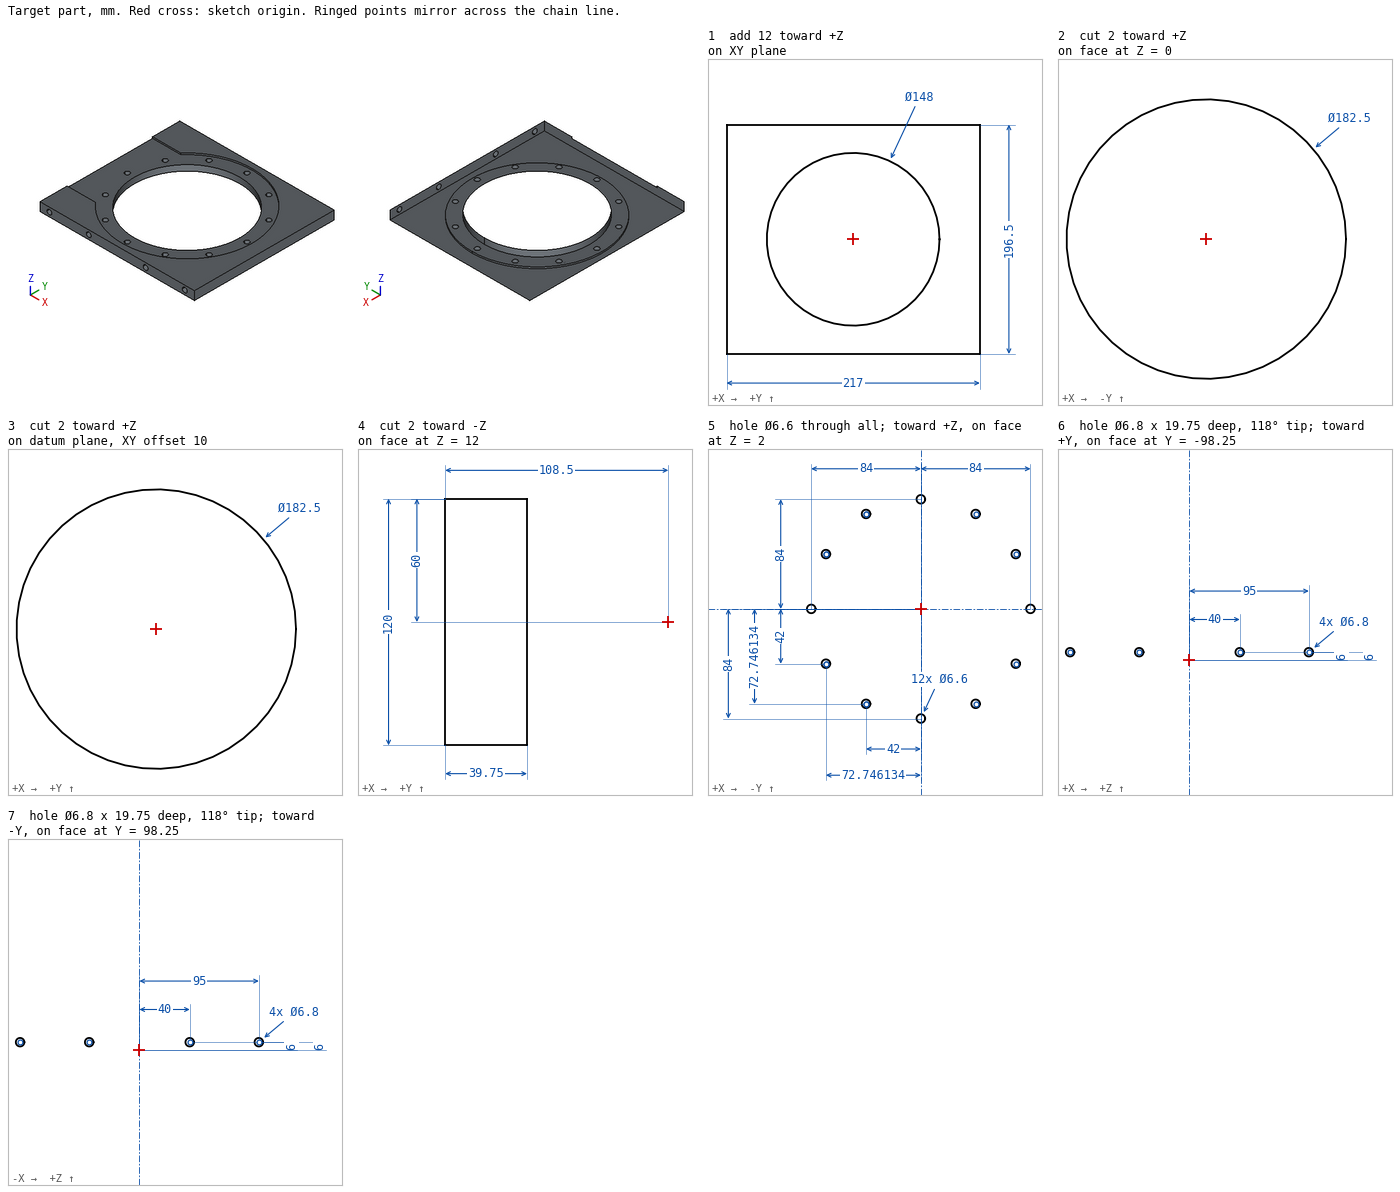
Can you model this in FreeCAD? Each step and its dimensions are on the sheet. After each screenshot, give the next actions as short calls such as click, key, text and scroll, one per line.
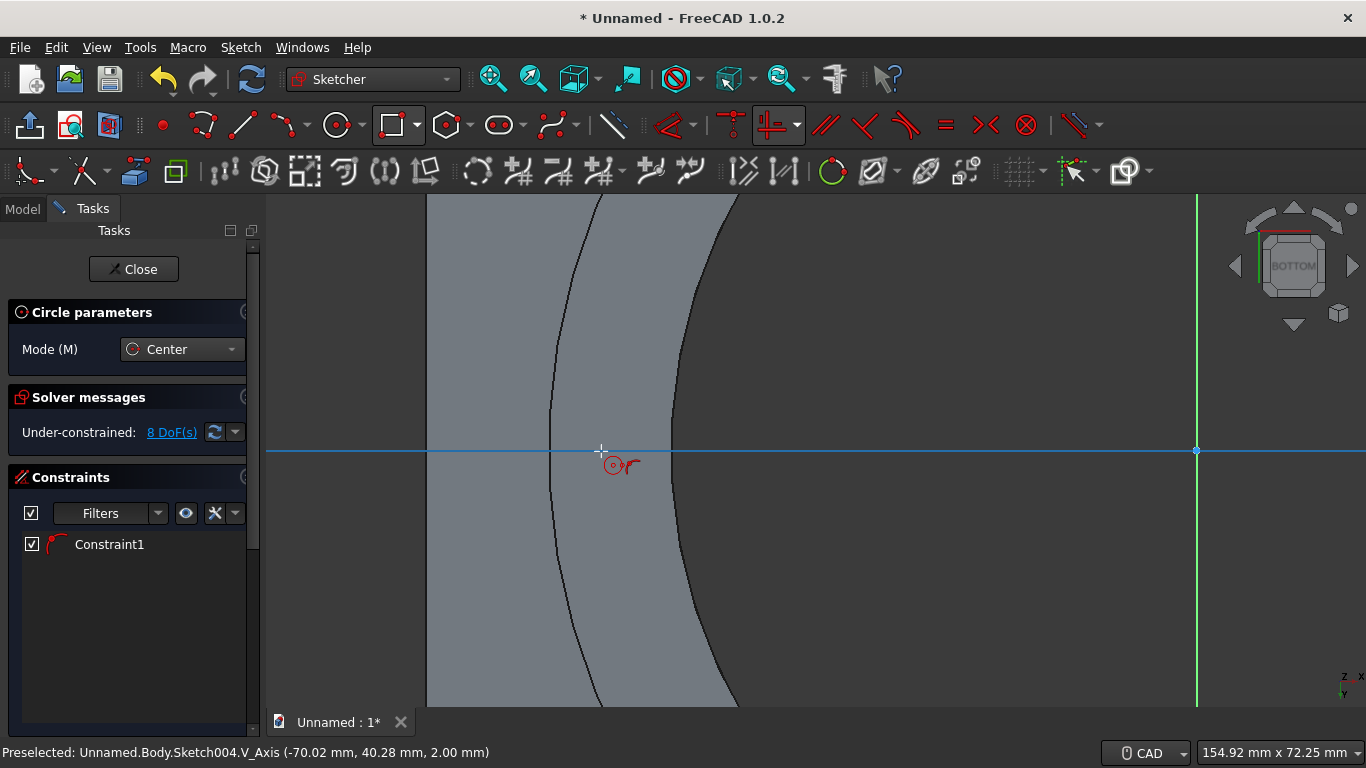
scroll(600, 450, down, 7)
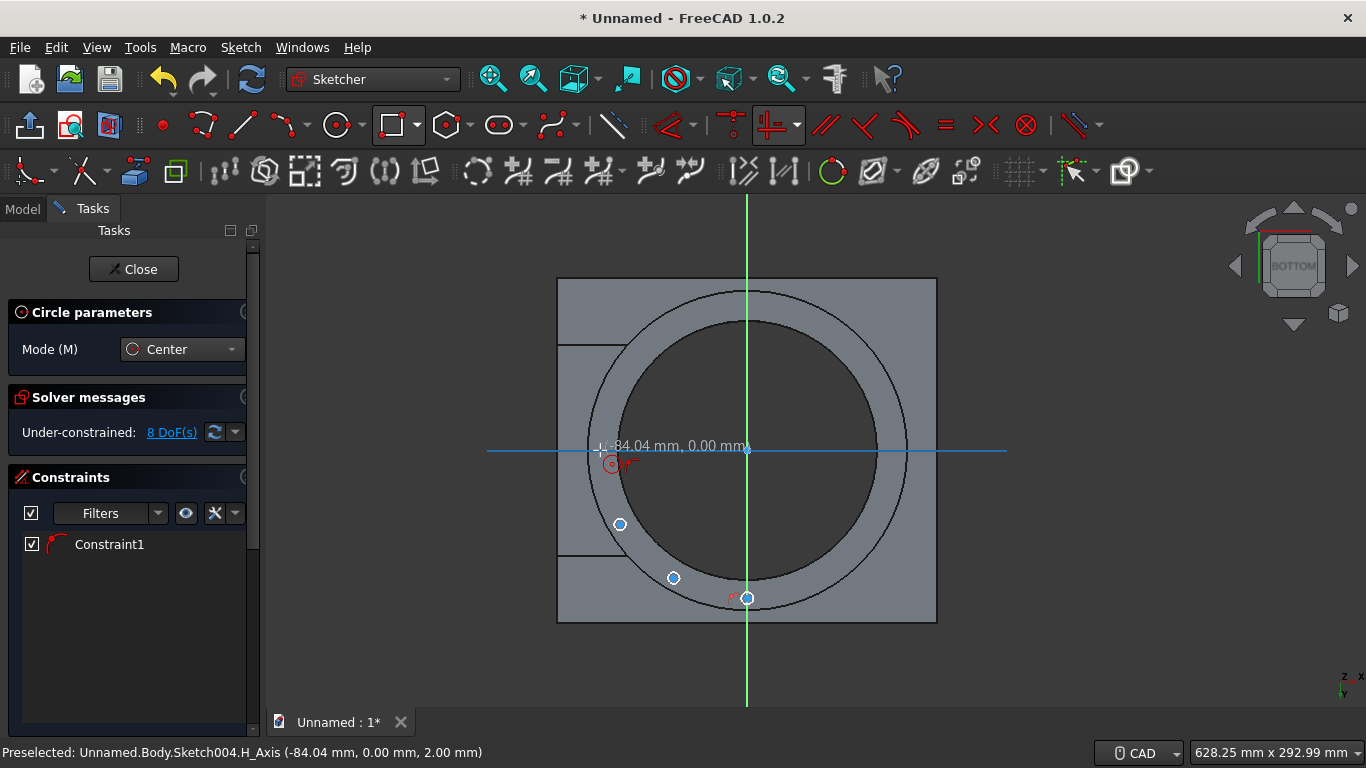
click(600, 451)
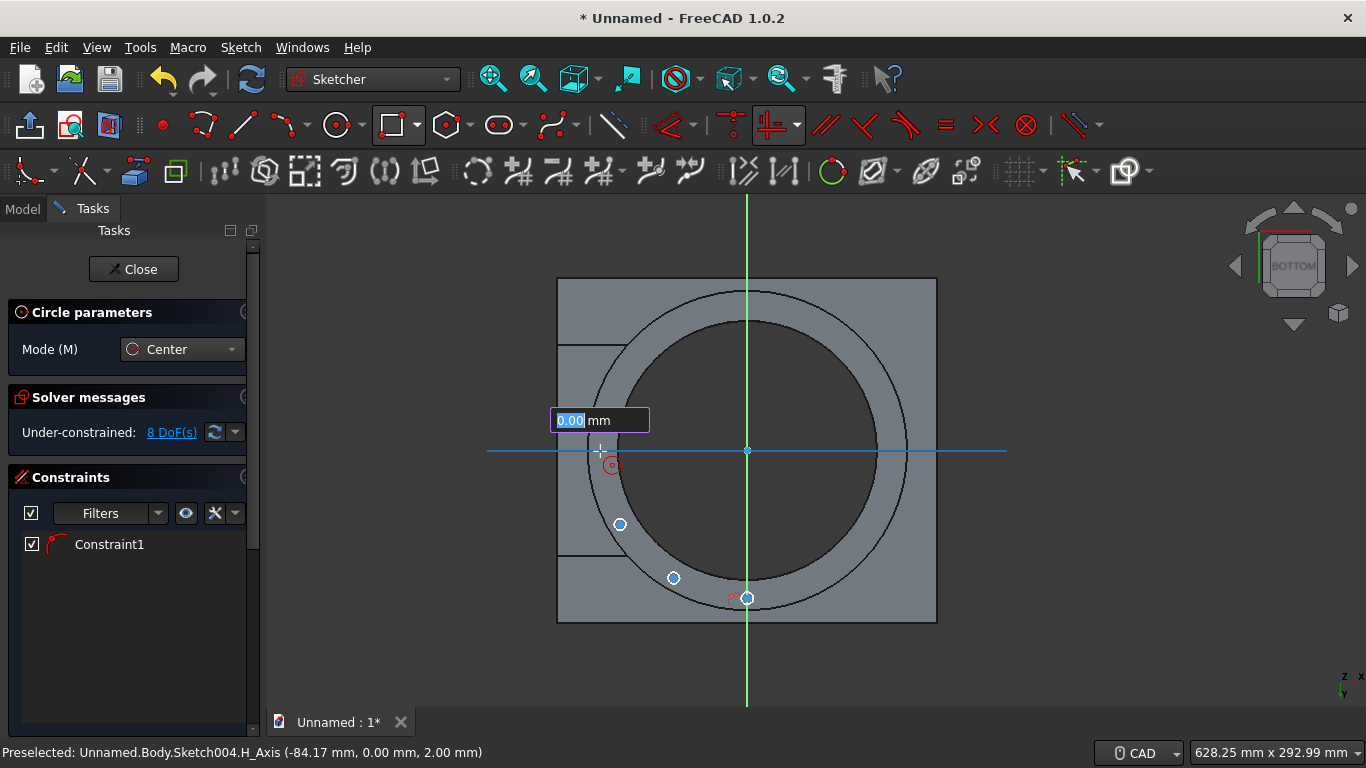
scroll(598, 456, up, 6)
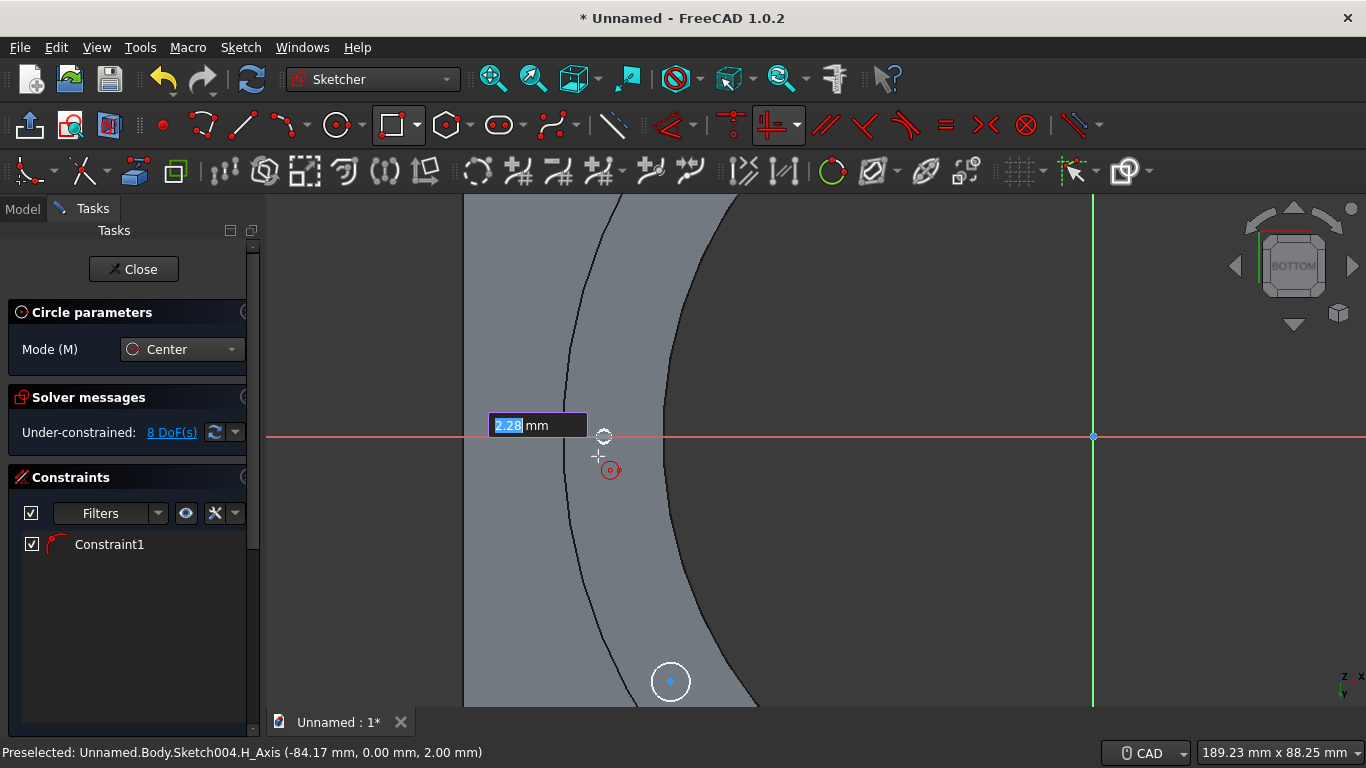
click(598, 455)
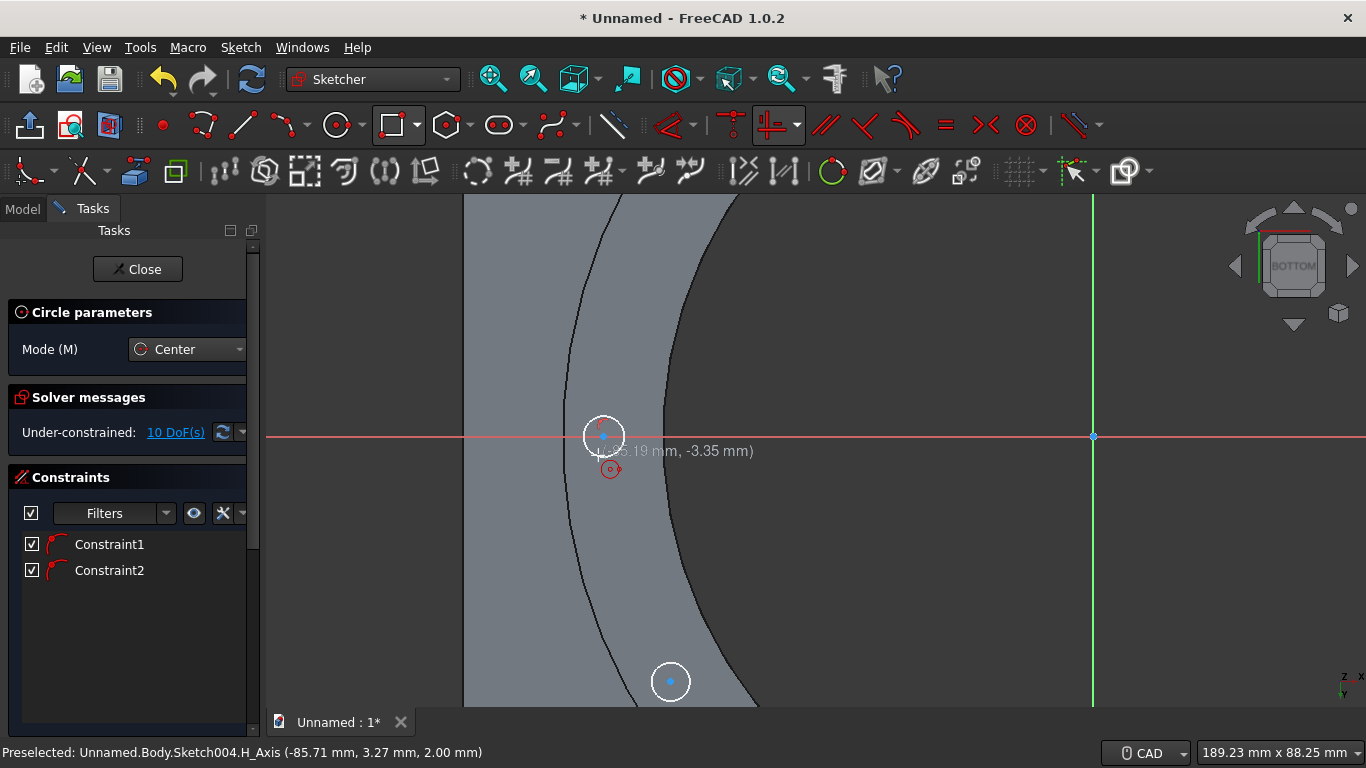
scroll(598, 457, down, 6)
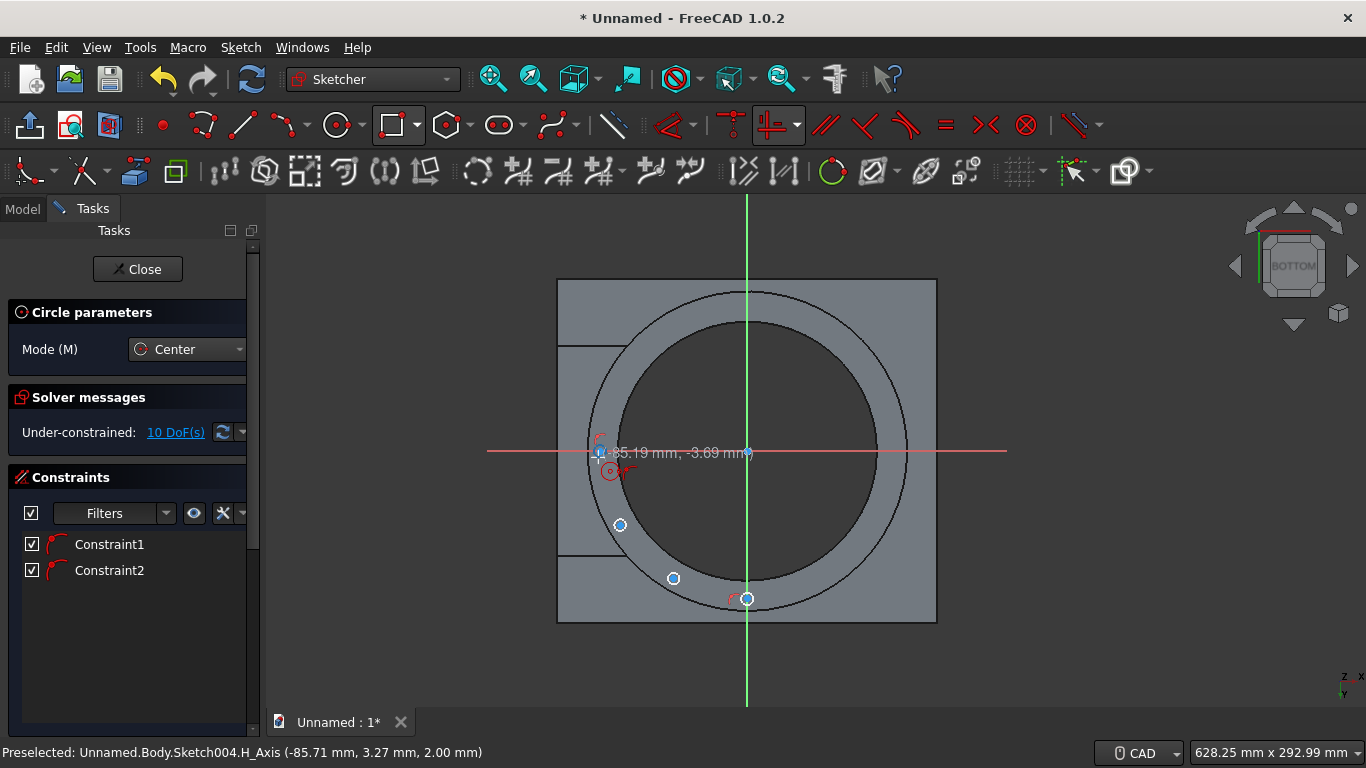
scroll(620, 378, up, 7)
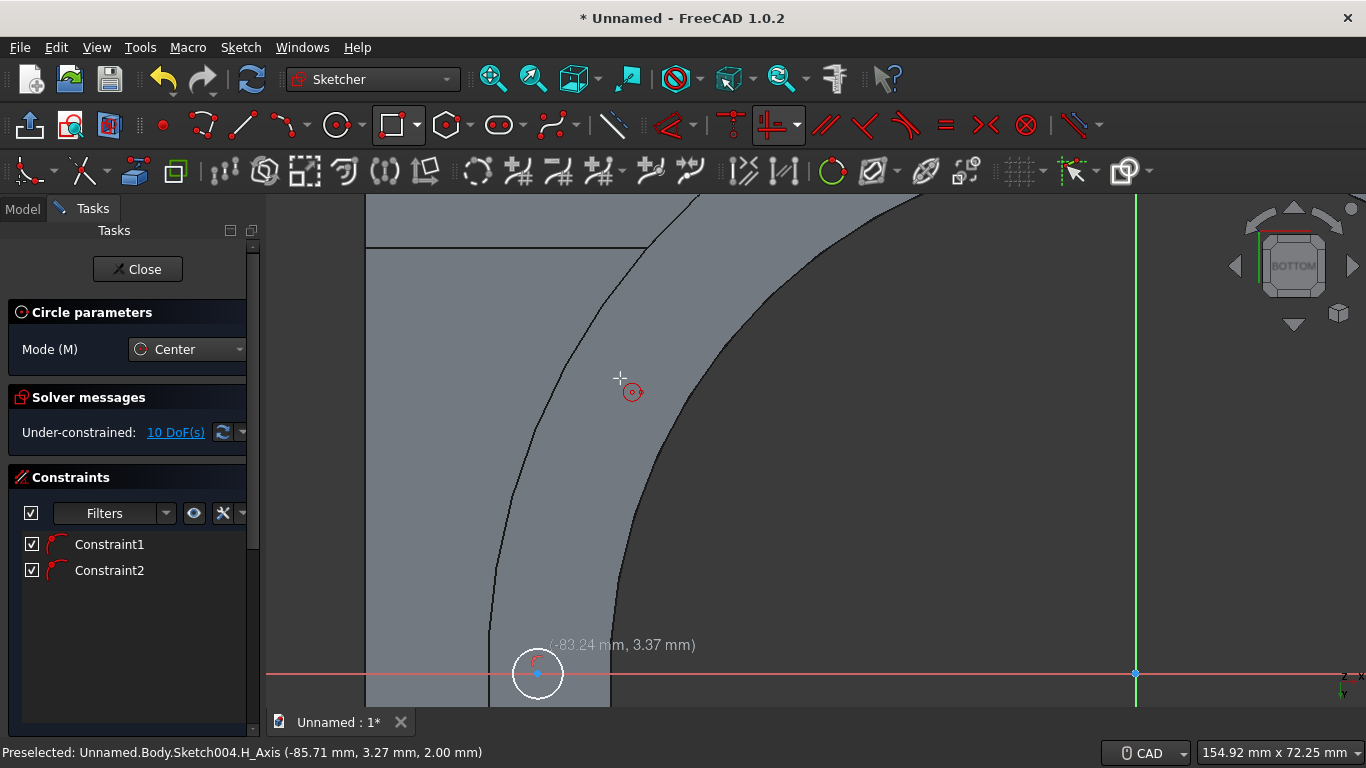
scroll(620, 377, down, 7)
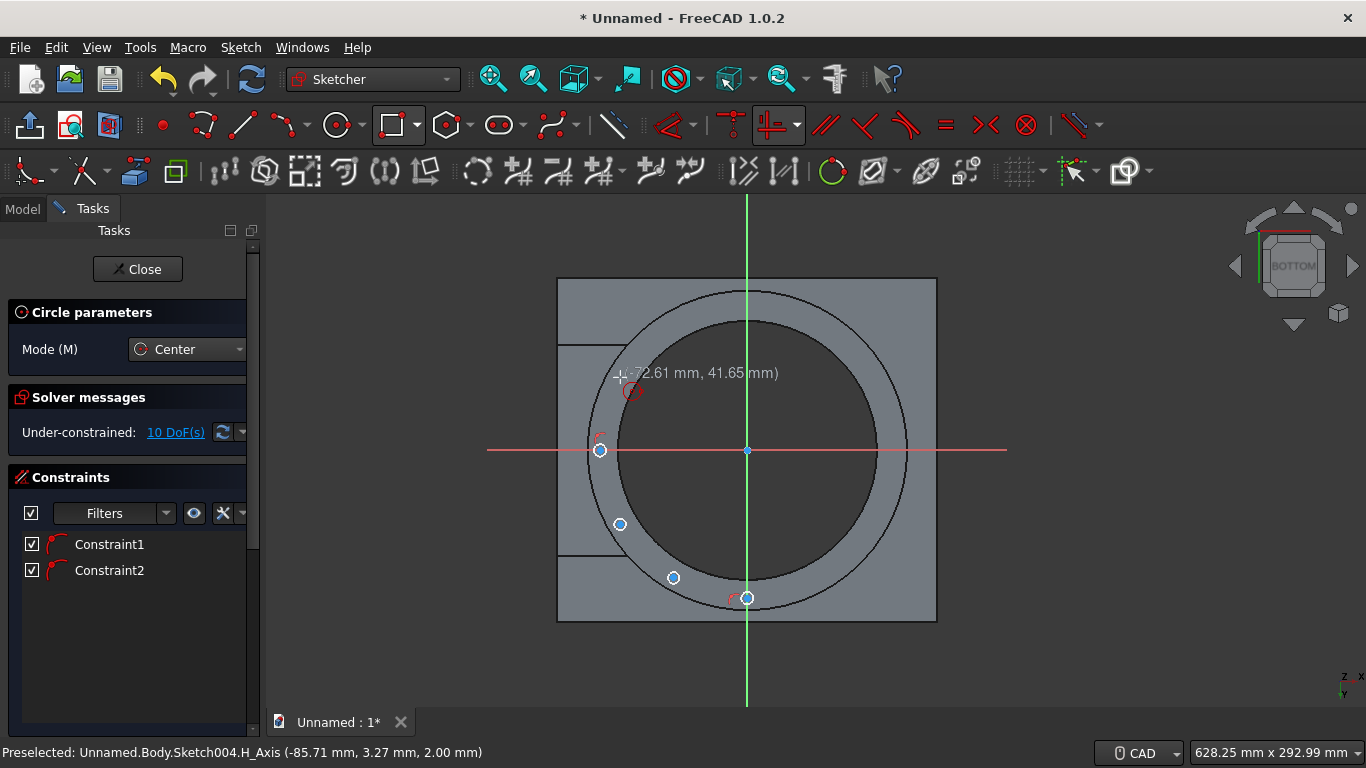
click(620, 377)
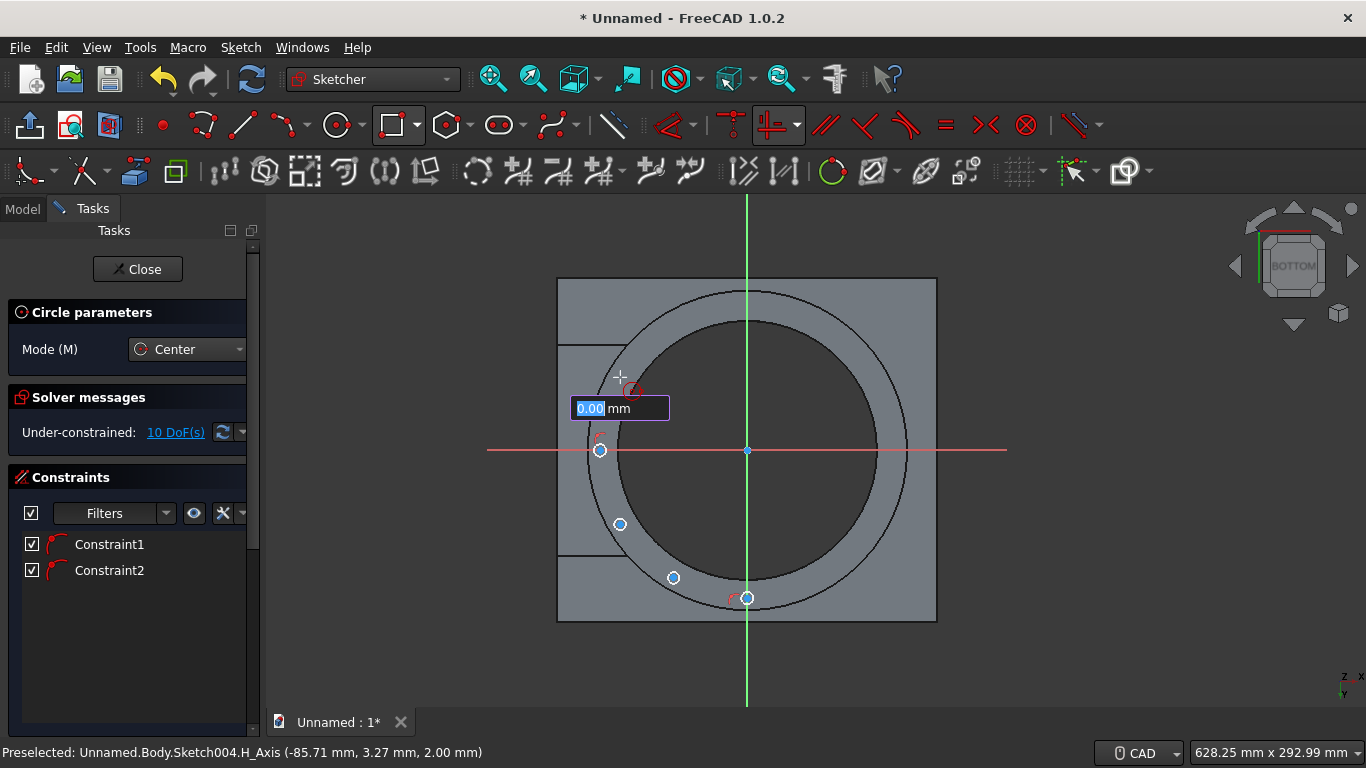
scroll(624, 373, up, 6)